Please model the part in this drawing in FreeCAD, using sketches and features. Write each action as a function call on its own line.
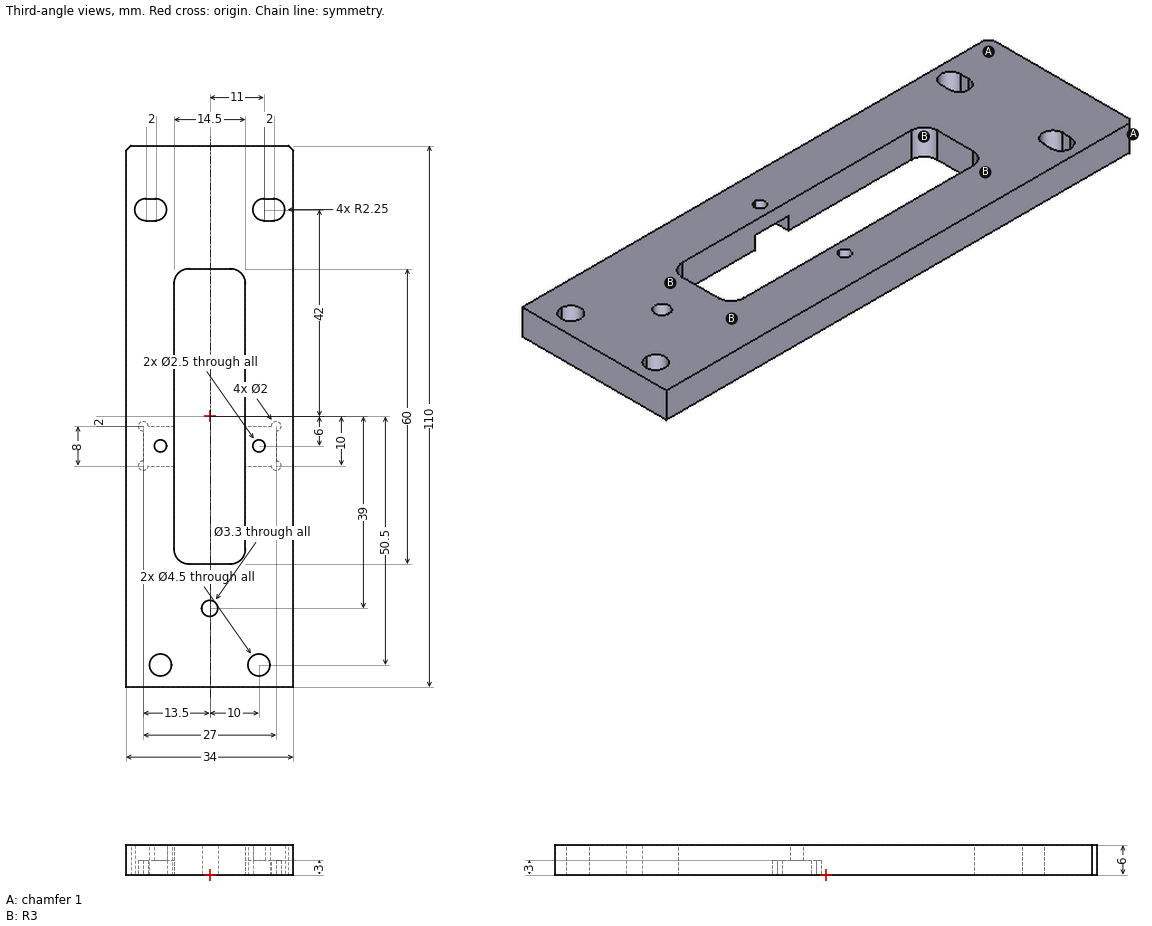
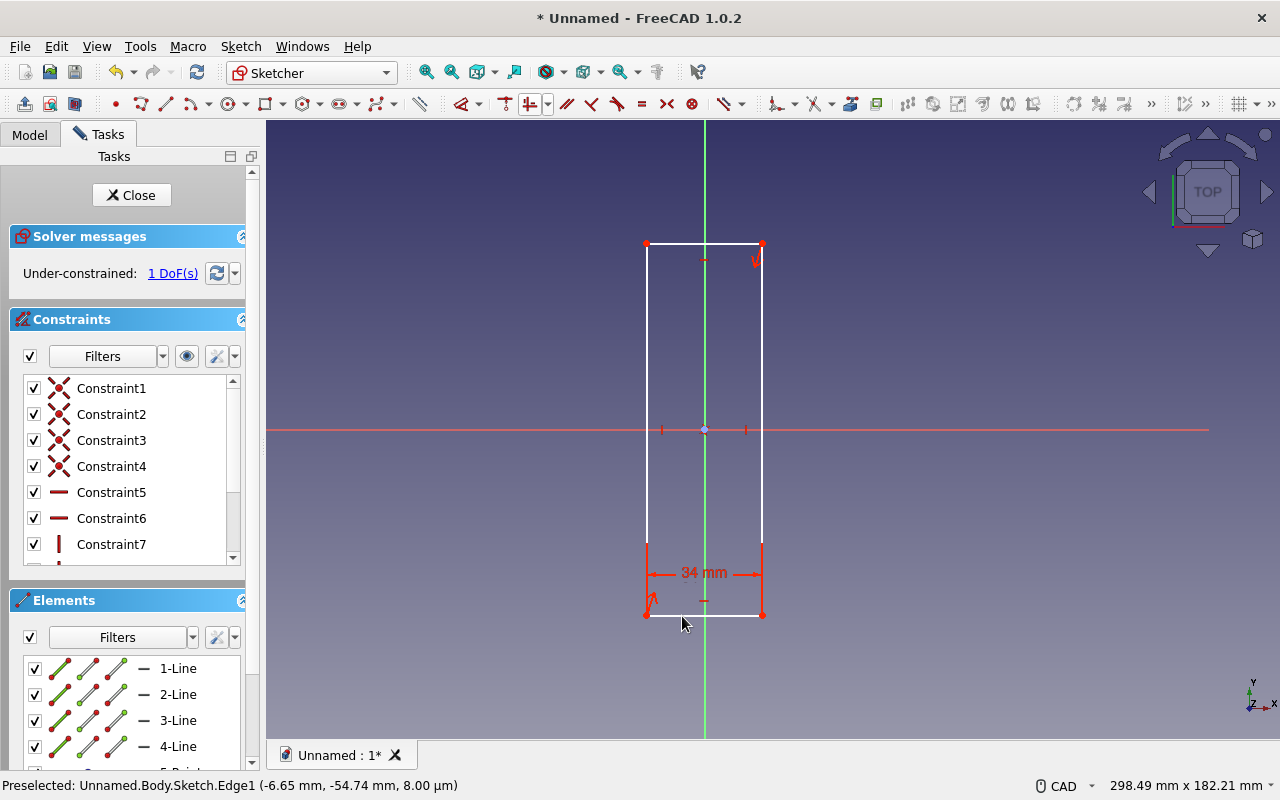
click(762, 504)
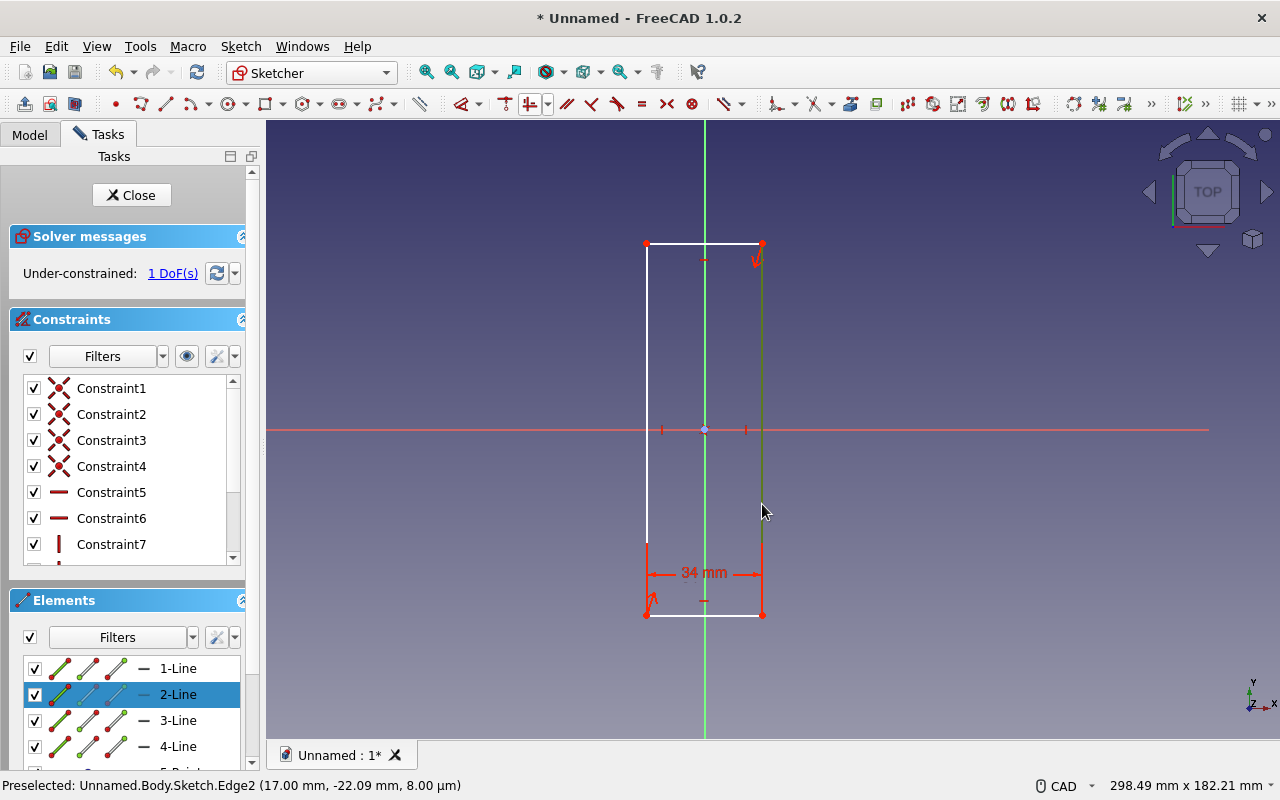
key(i)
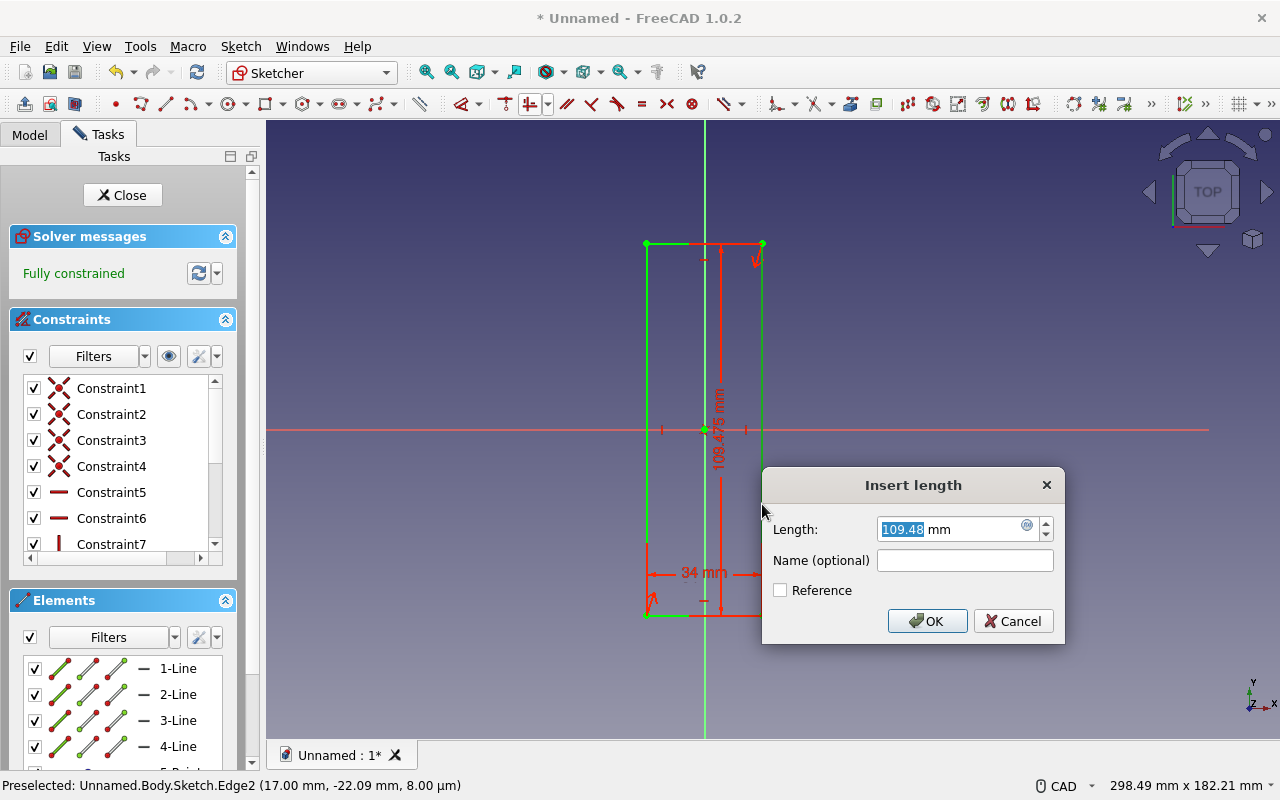
text(110)
key(Return)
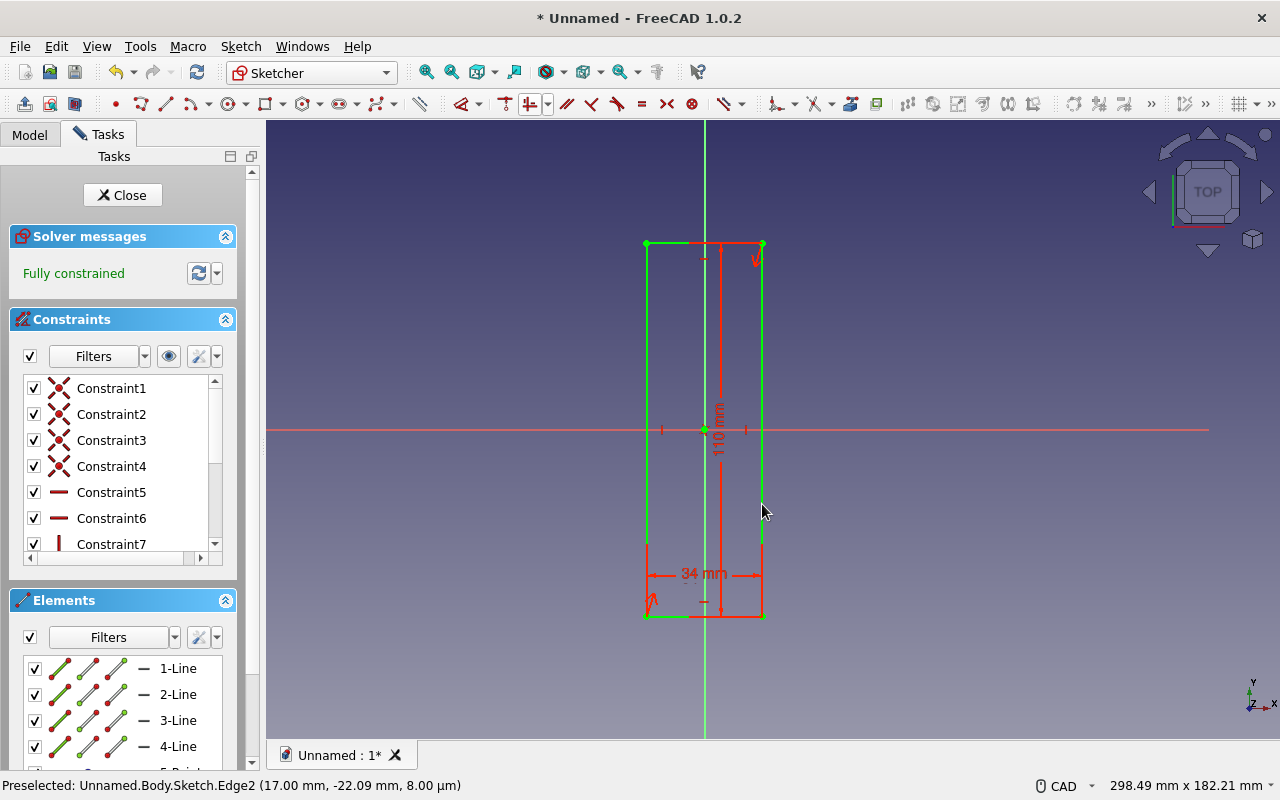
click(123, 195)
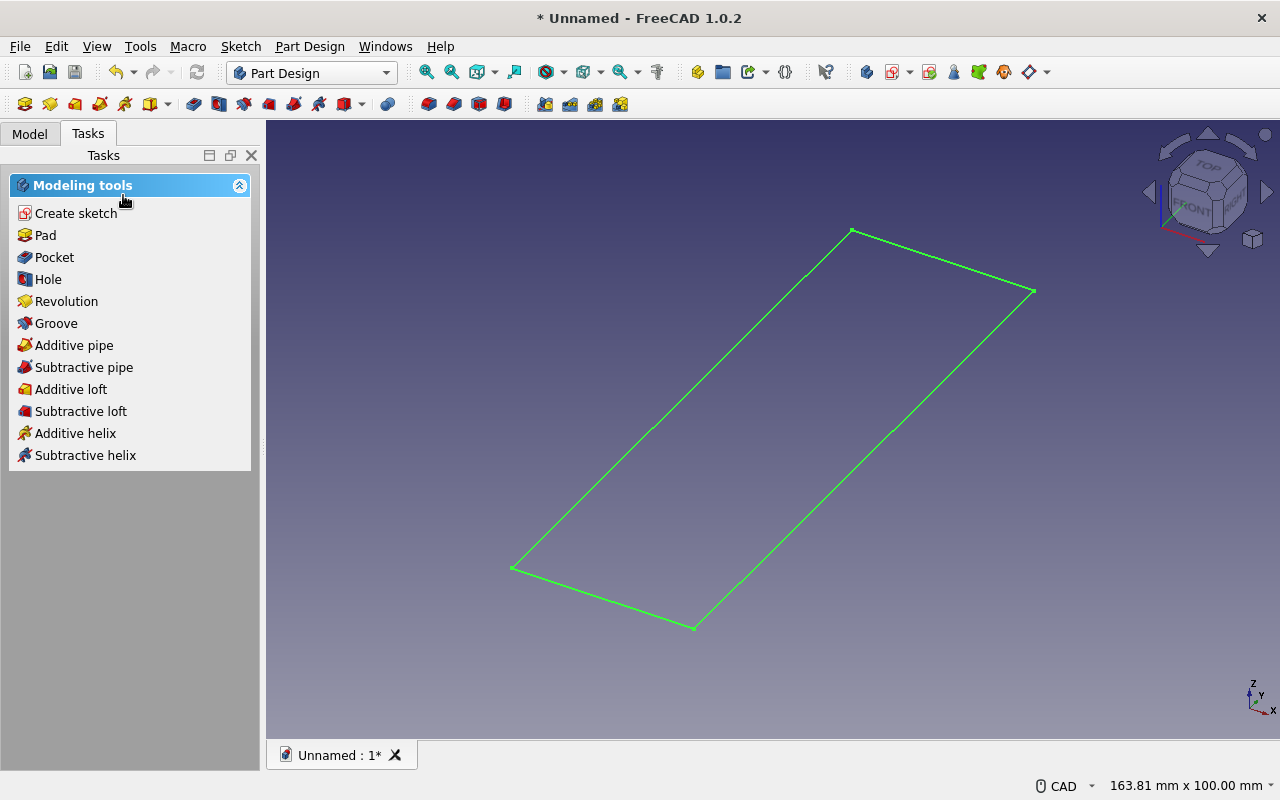
click(25, 104)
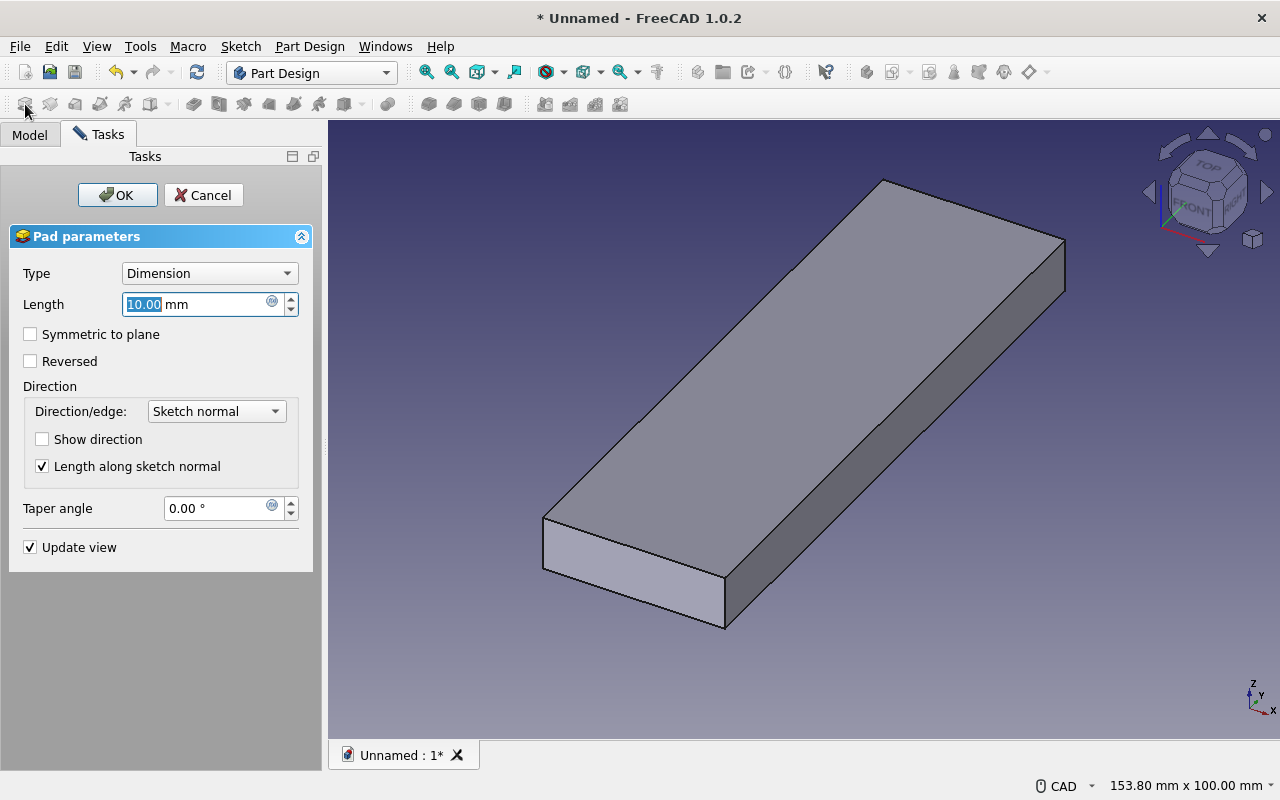
text(6)
key(Tab)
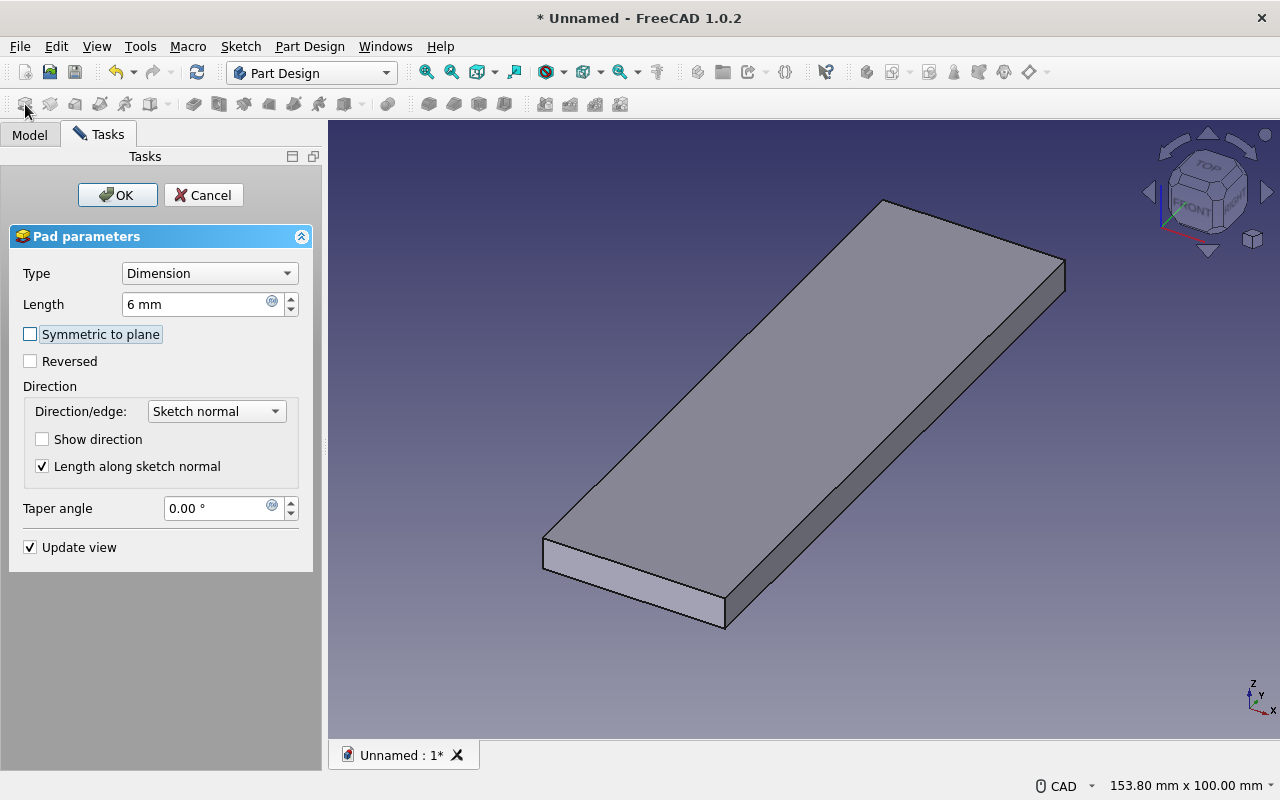
click(118, 195)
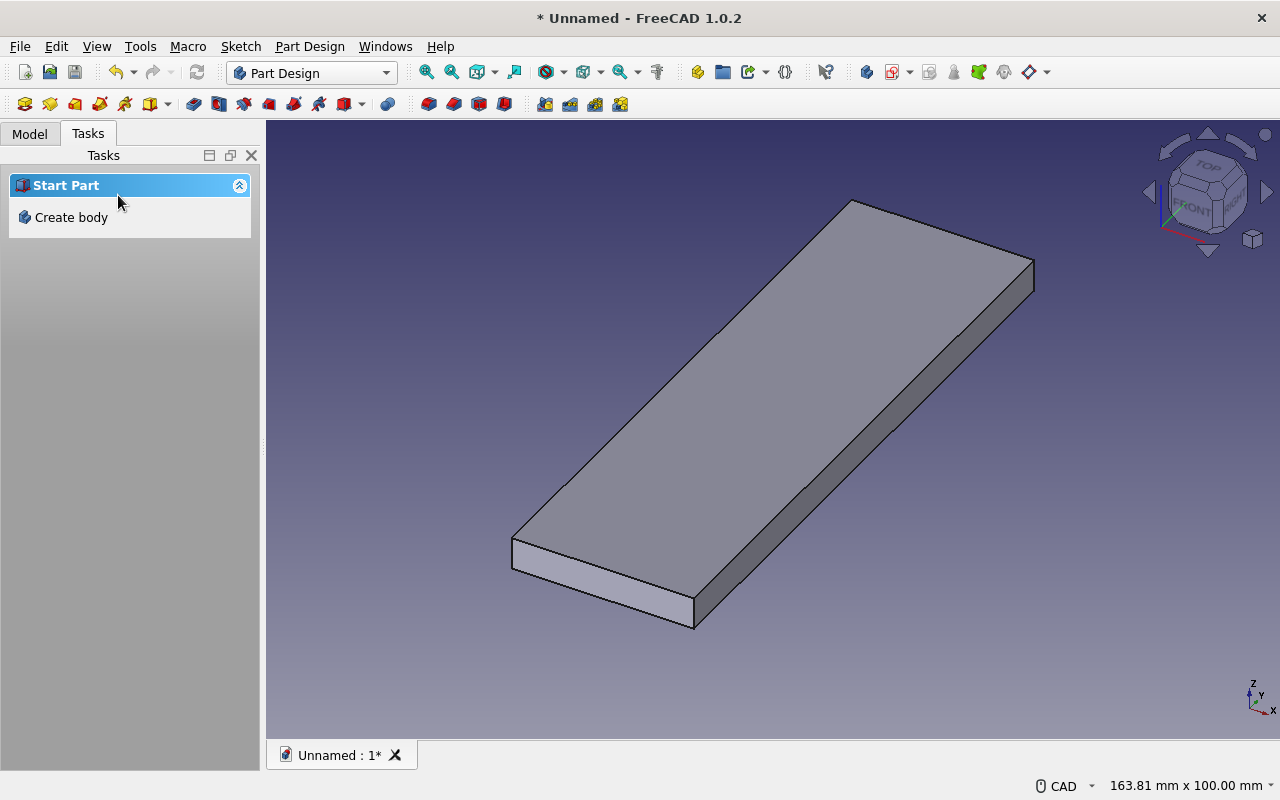
key(0)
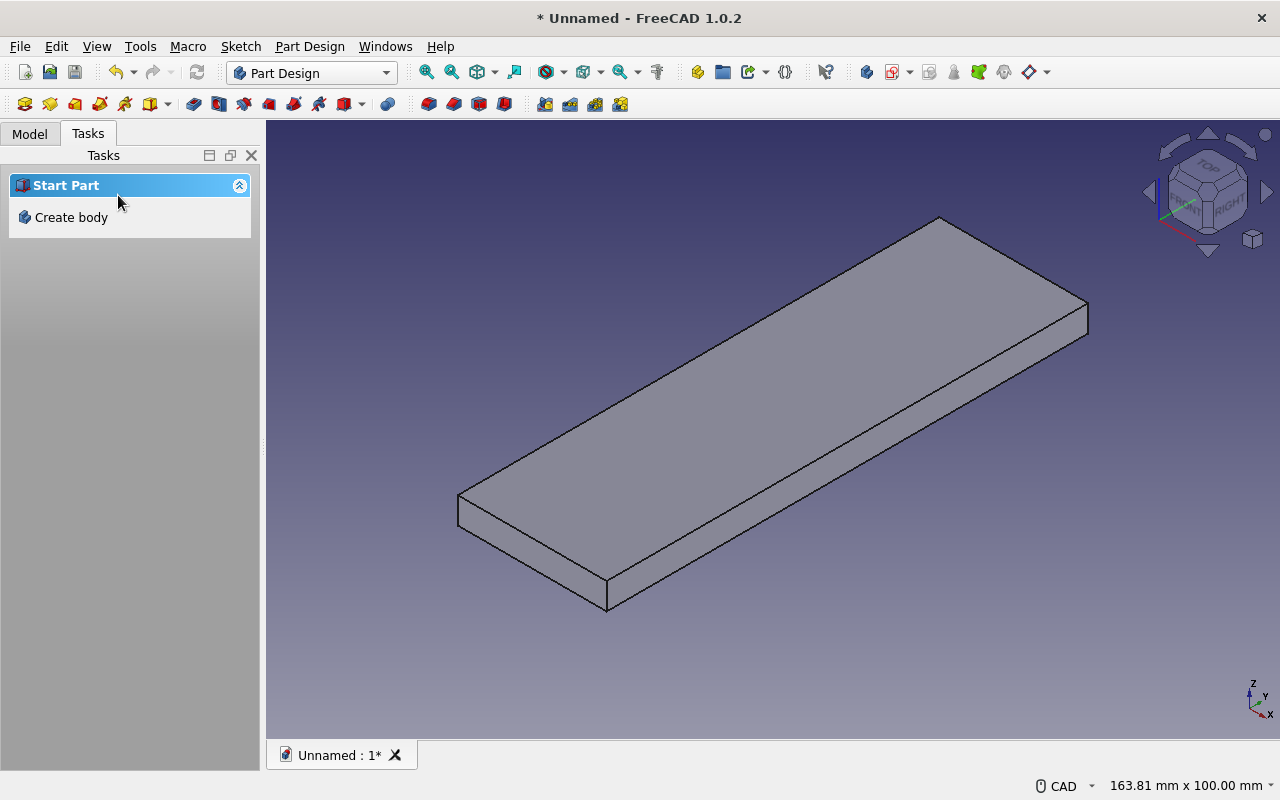
key(2)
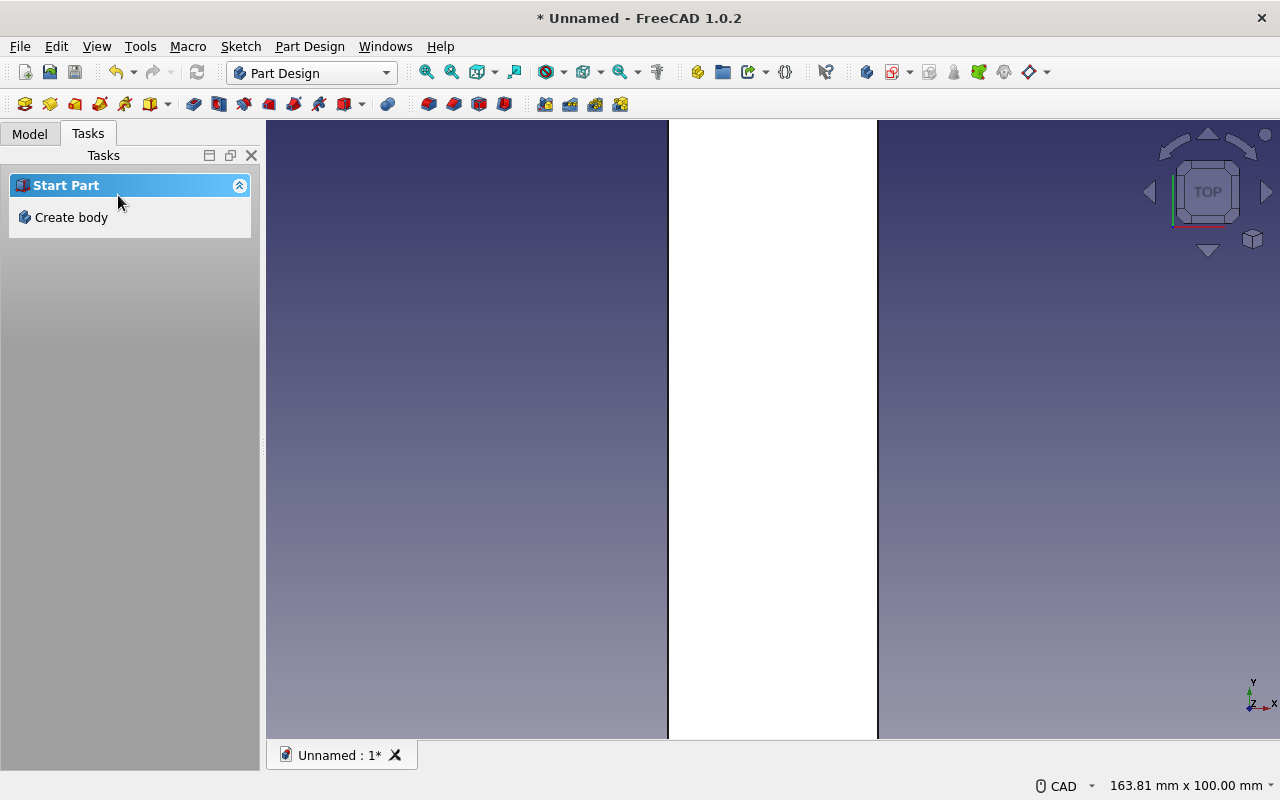
key(v)
key(f)